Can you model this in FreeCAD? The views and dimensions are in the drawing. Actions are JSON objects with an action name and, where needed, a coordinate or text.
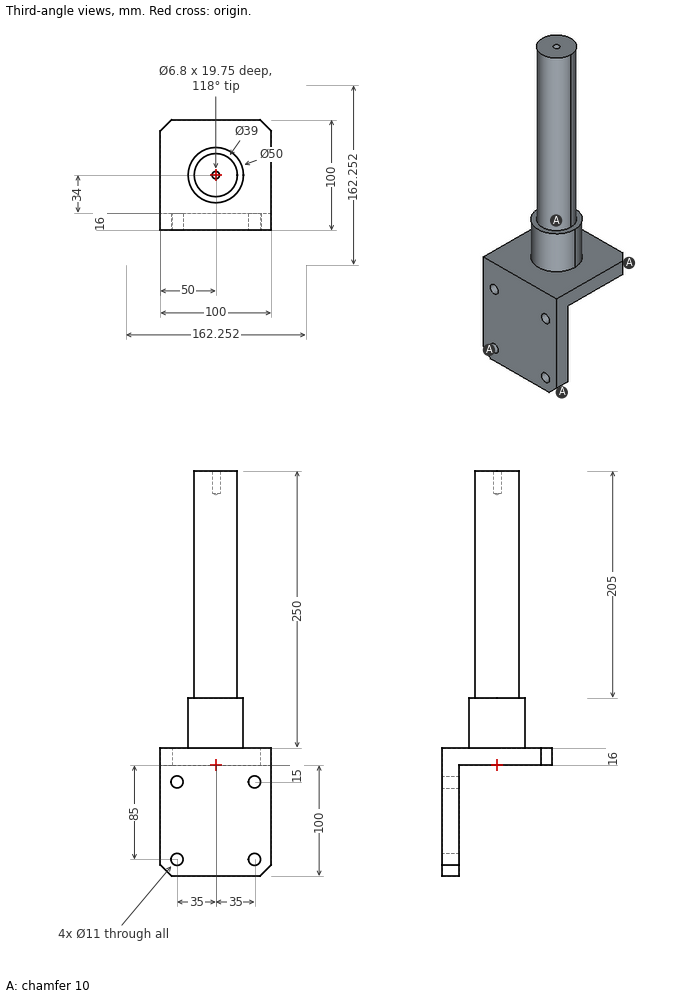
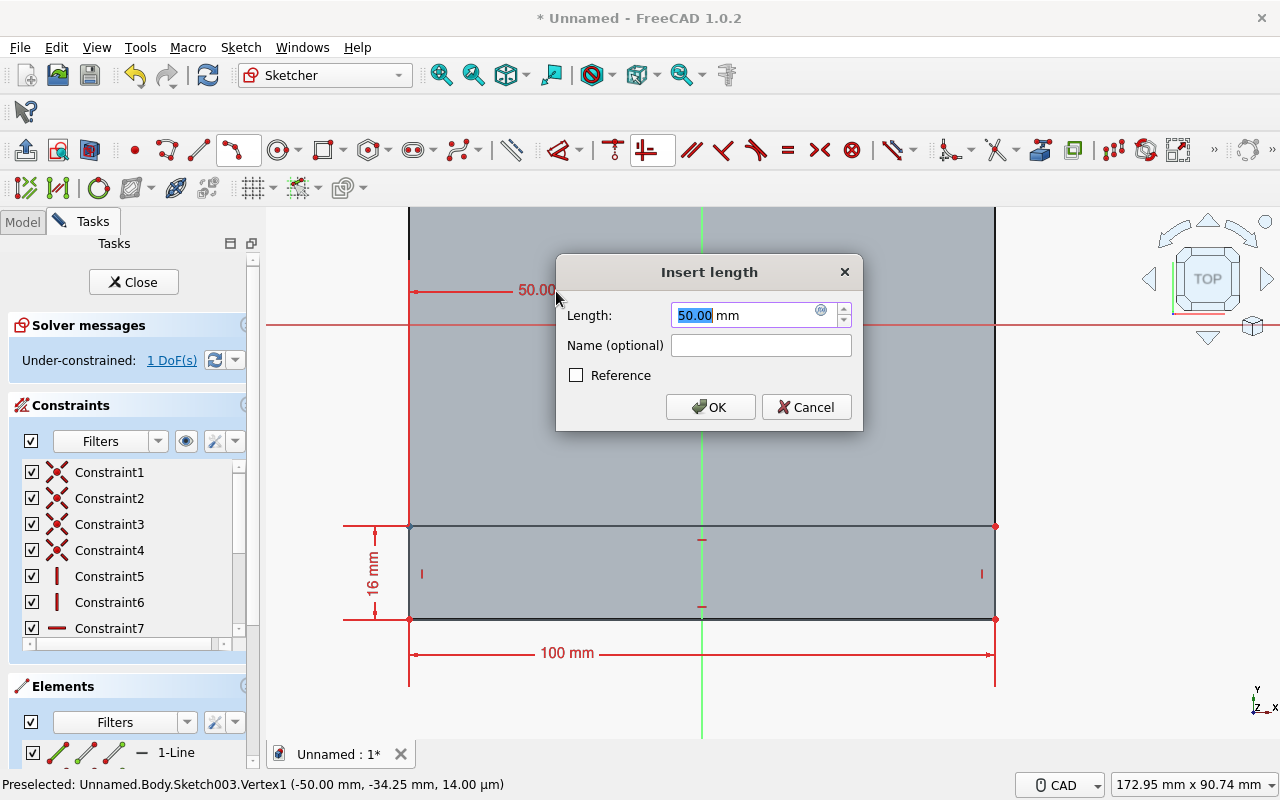
{"action": "type", "text": "50"}
{"action": "key", "text": "Return"}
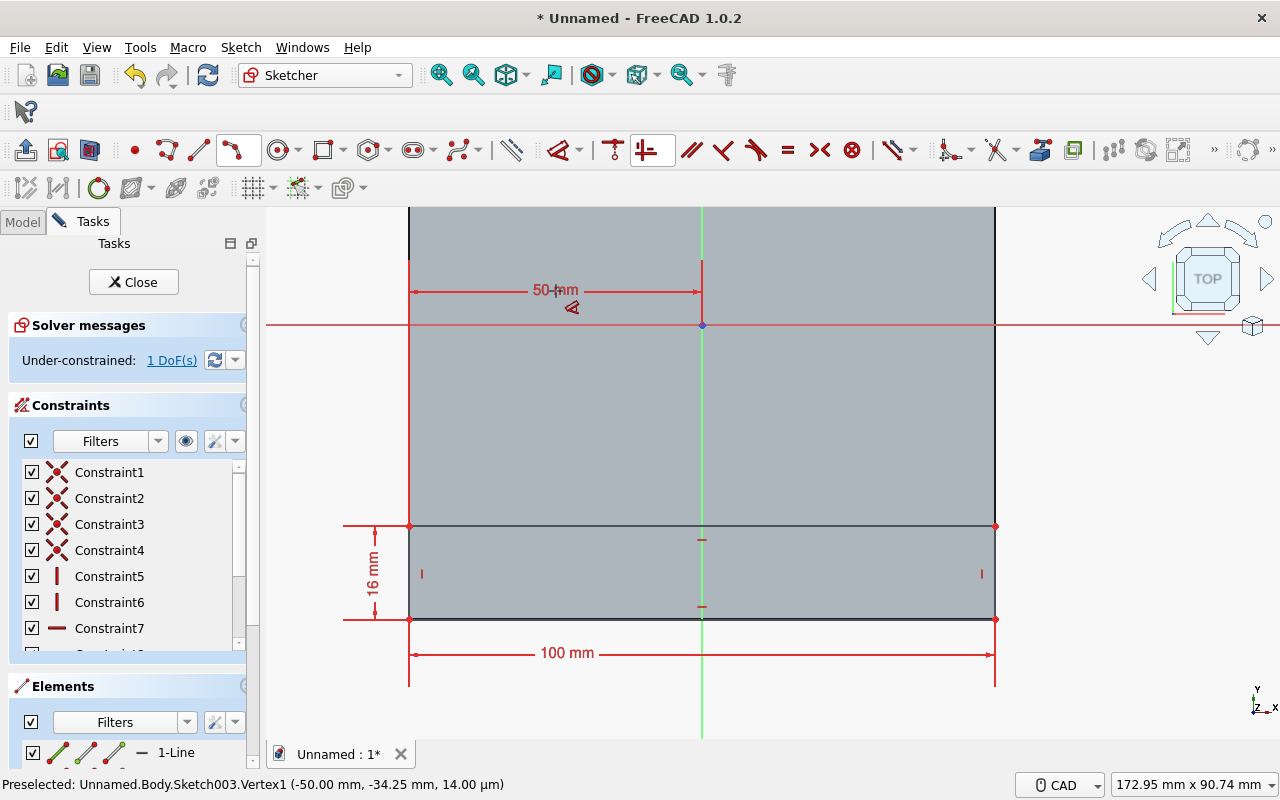
{"action": "left_click", "coordinate": [409, 526]}
{"action": "left_click", "coordinate": [375, 426]}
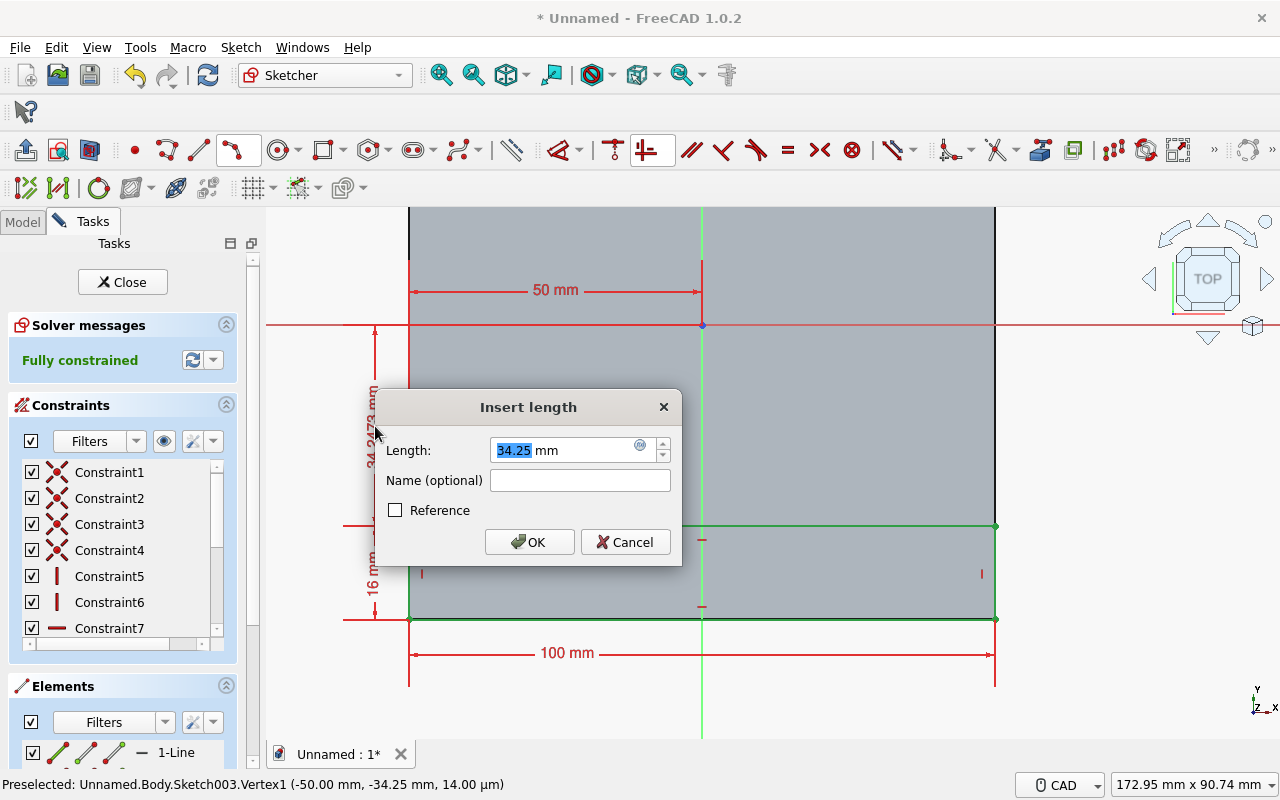
{"action": "type", "text": "34"}
{"action": "key", "text": "Return"}
{"action": "key", "text": "Escape"}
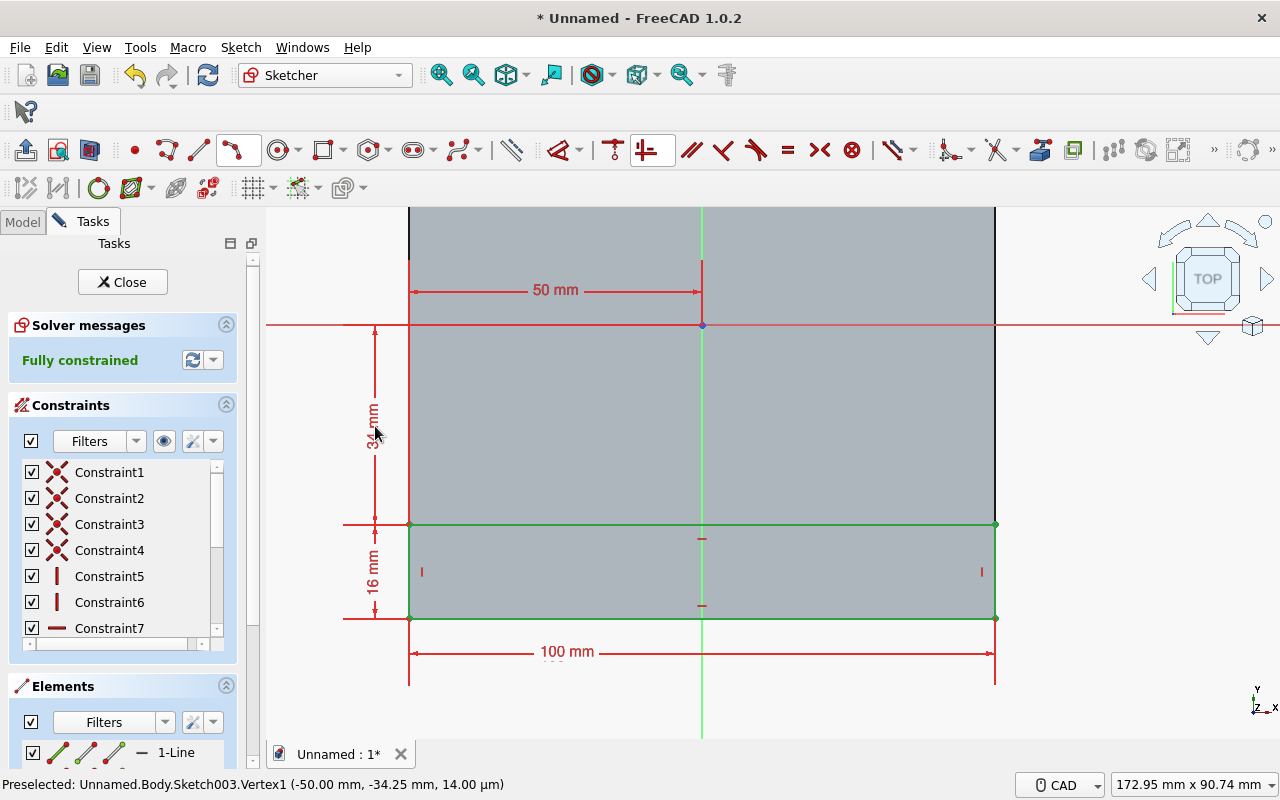
{"action": "left_click", "coordinate": [123, 282]}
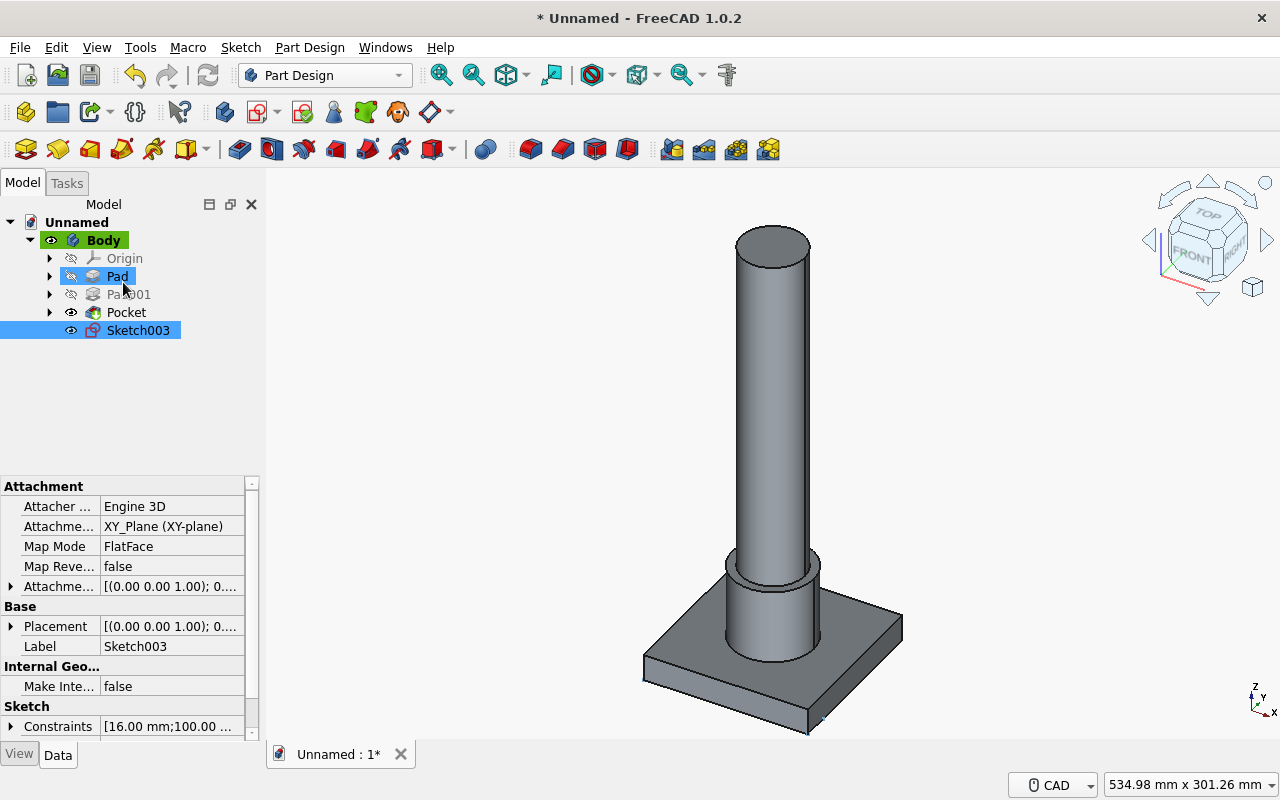
{"action": "left_click", "coordinate": [26, 150]}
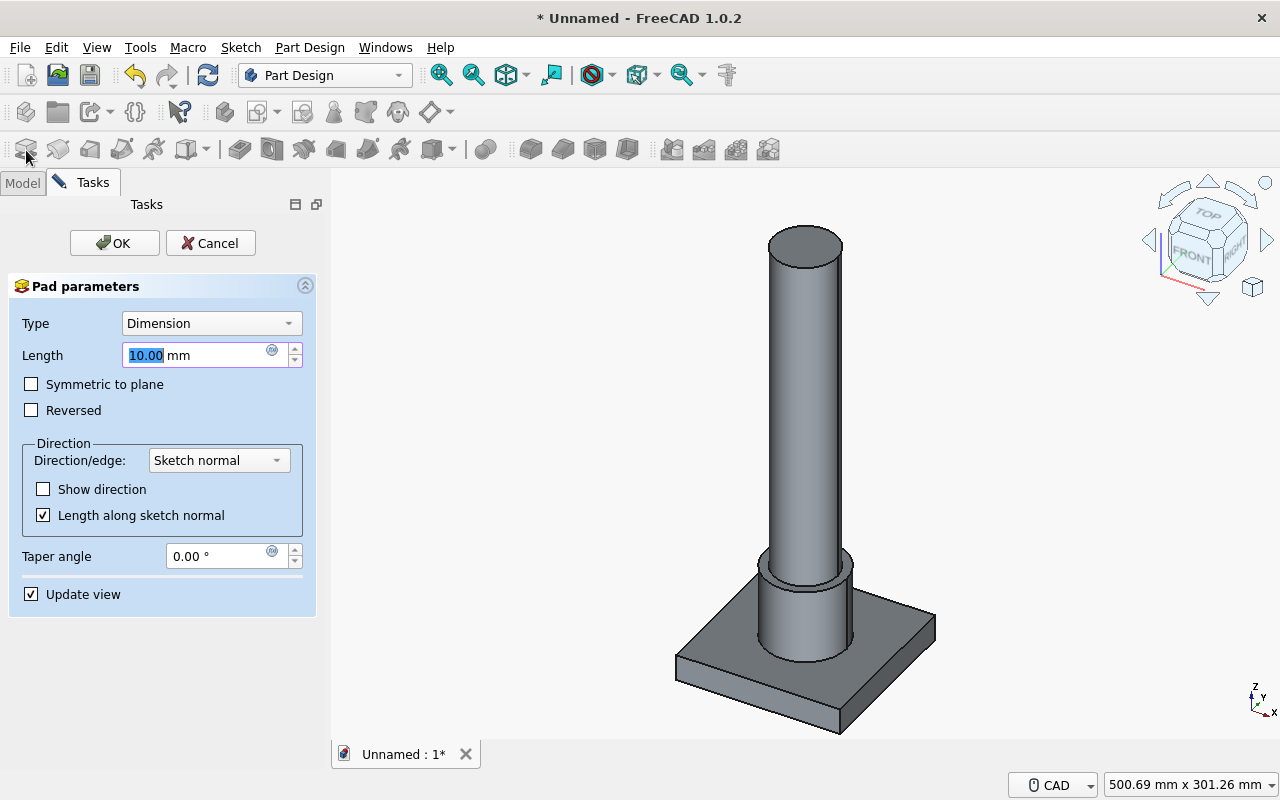
{"action": "type", "text": "100"}
{"action": "key", "text": "Tab"}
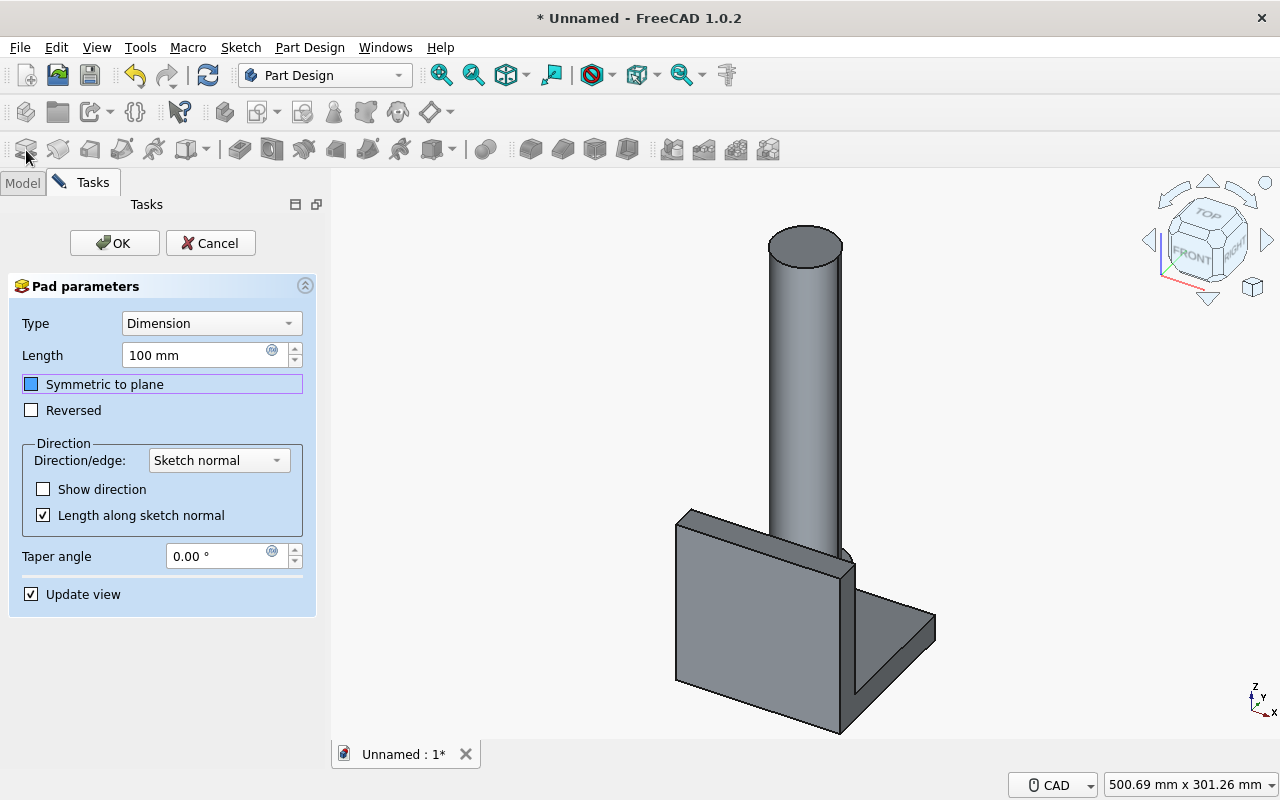
{"action": "left_click", "coordinate": [30, 410]}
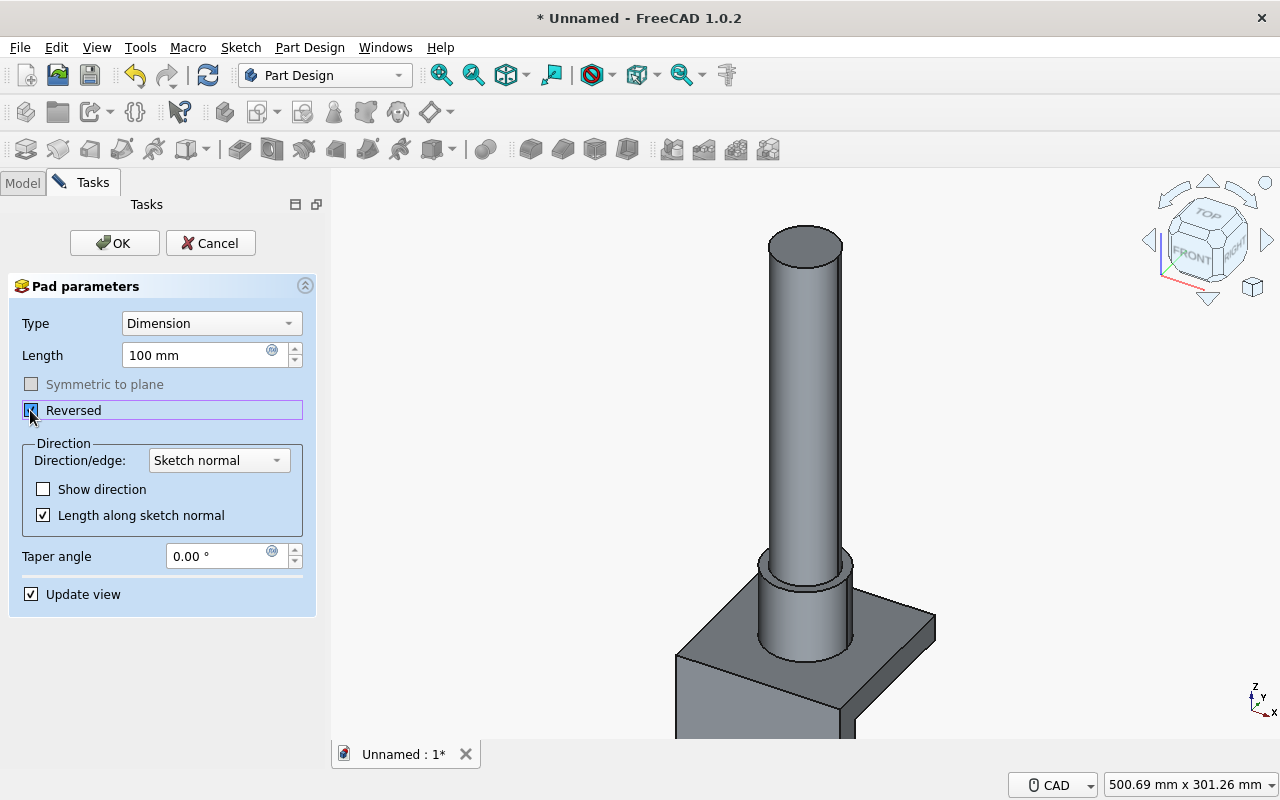
{"action": "left_click", "coordinate": [115, 243]}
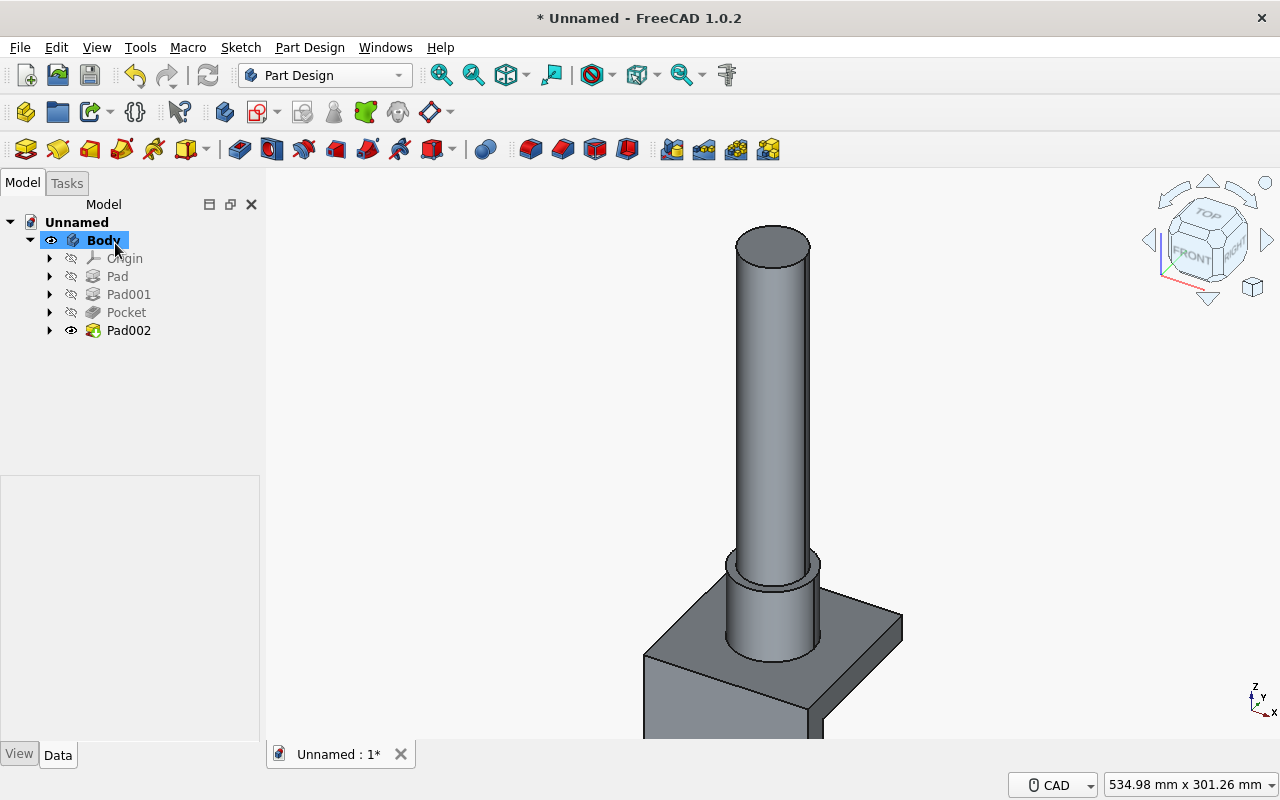
{"action": "left_click", "coordinate": [442, 76]}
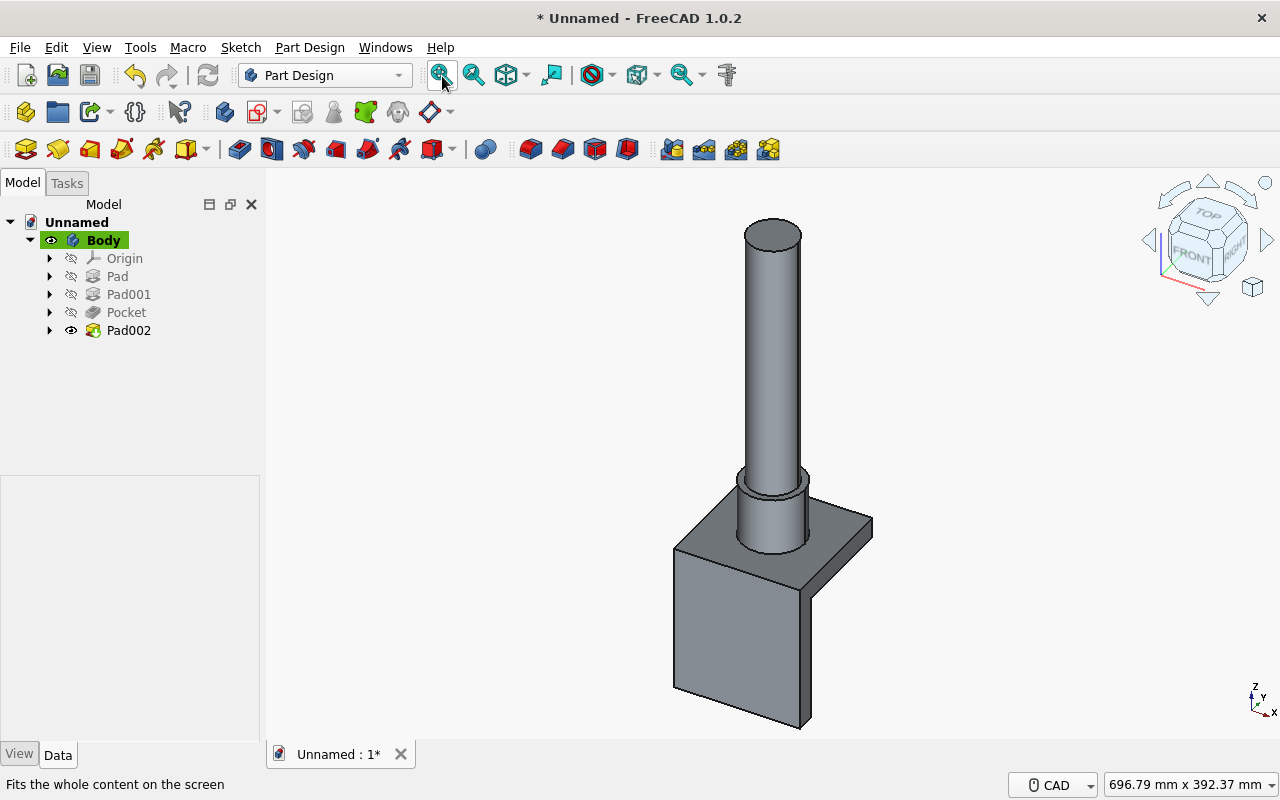
{"action": "left_click", "coordinate": [773, 234]}